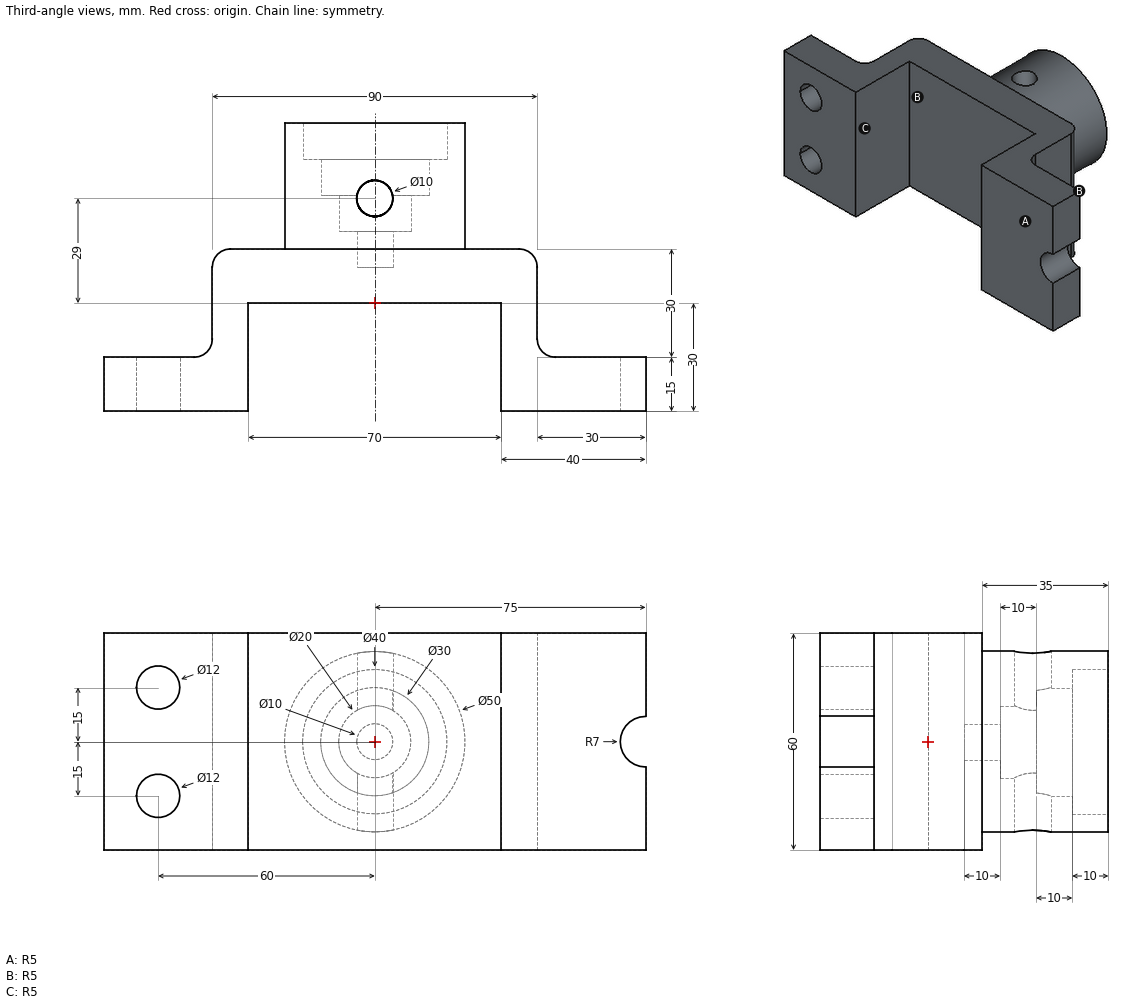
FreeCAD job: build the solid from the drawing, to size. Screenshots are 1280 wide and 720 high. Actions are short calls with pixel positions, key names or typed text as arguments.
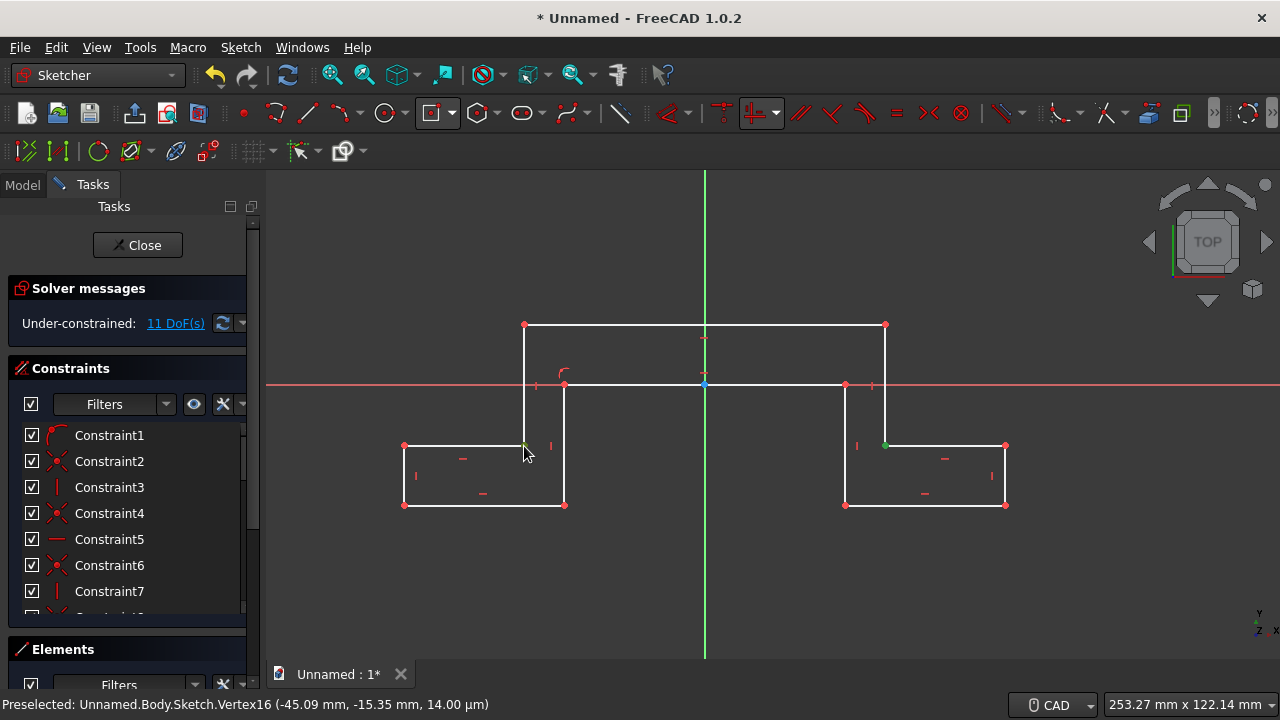
click(705, 600)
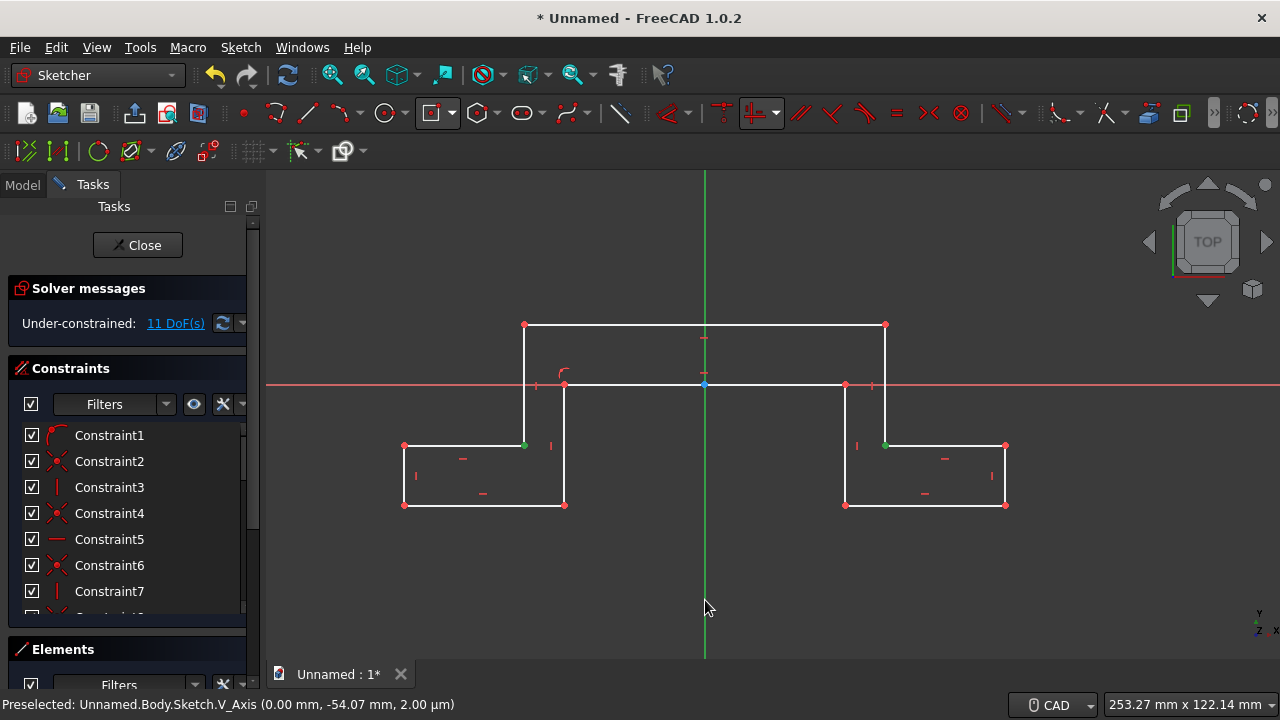
click(930, 114)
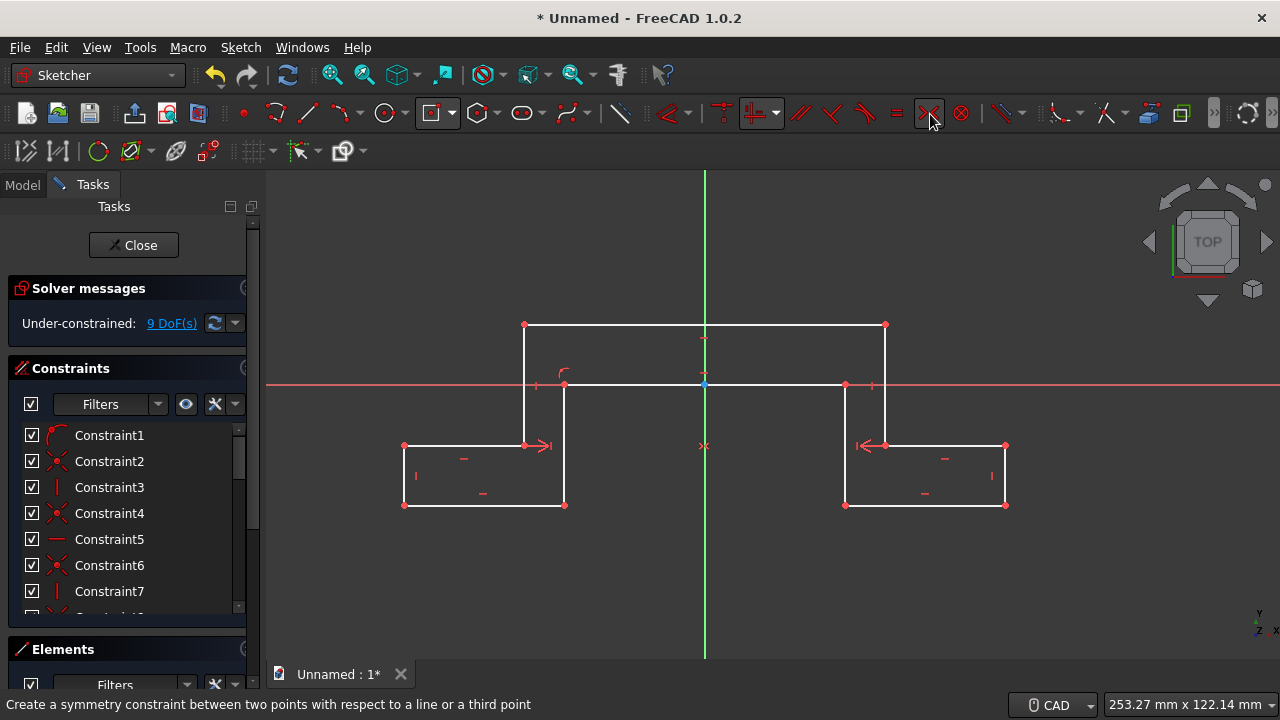
click(1005, 506)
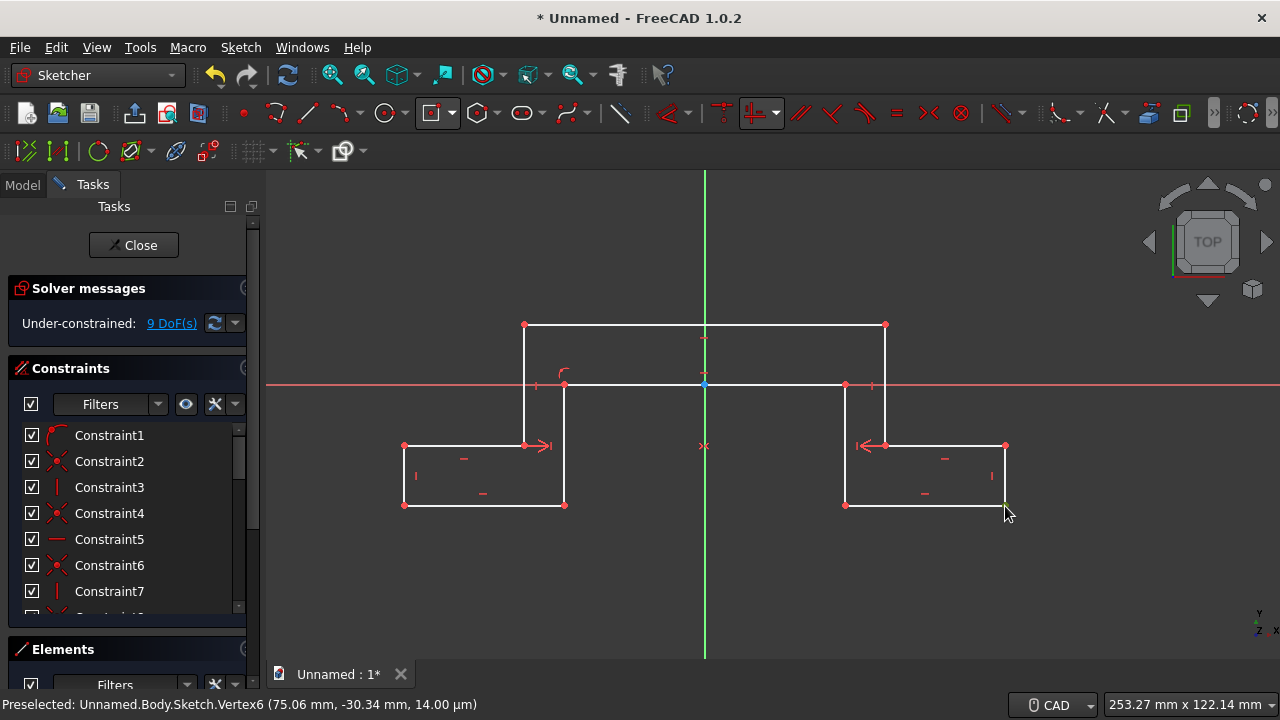
click(404, 506)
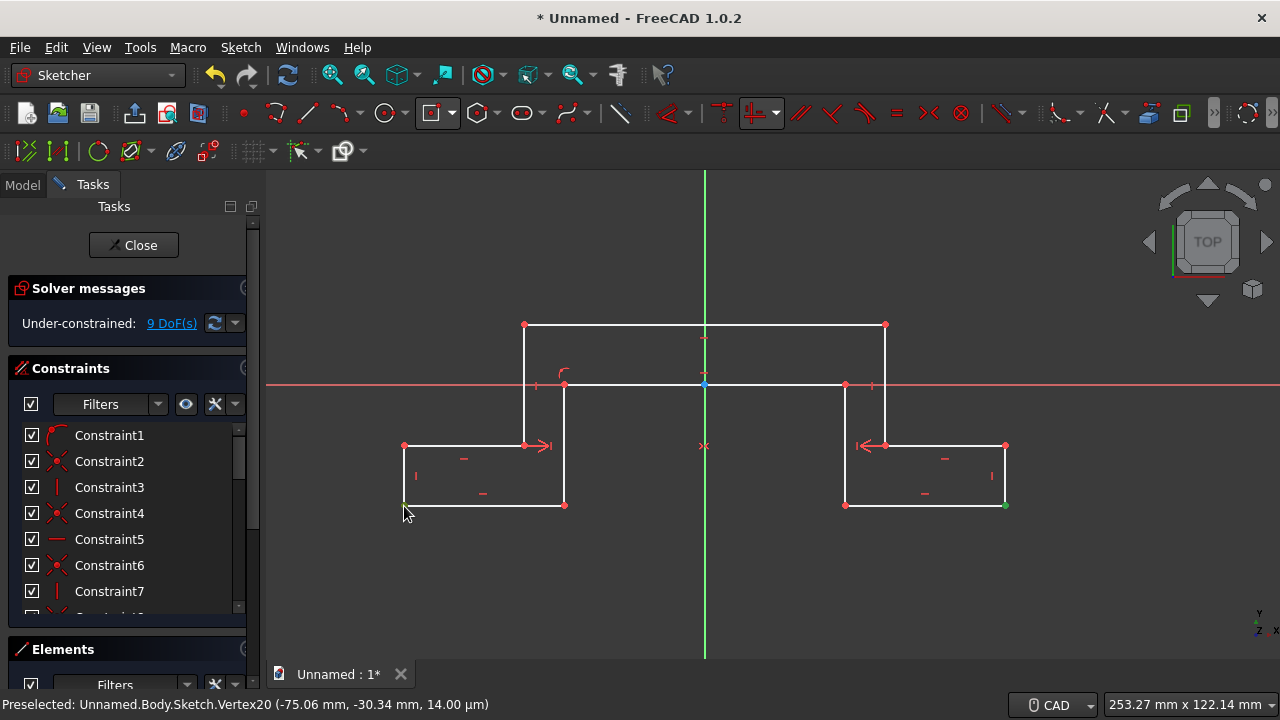
click(705, 600)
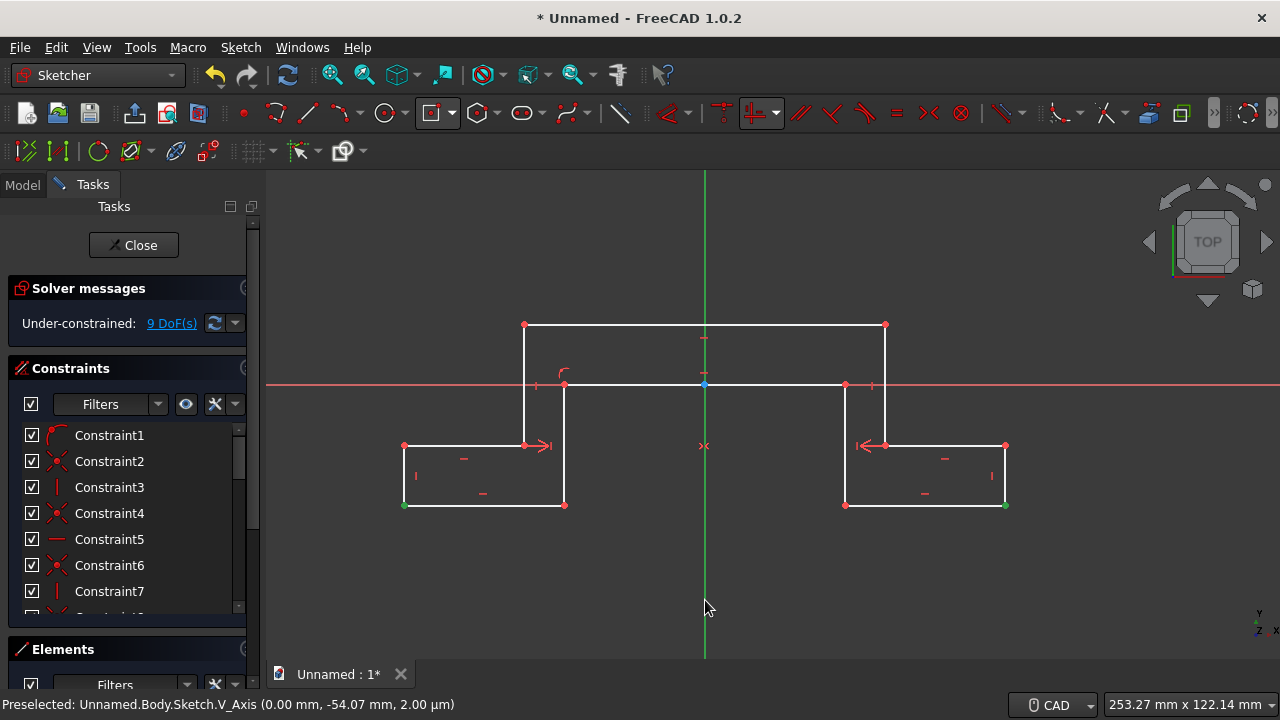
click(930, 114)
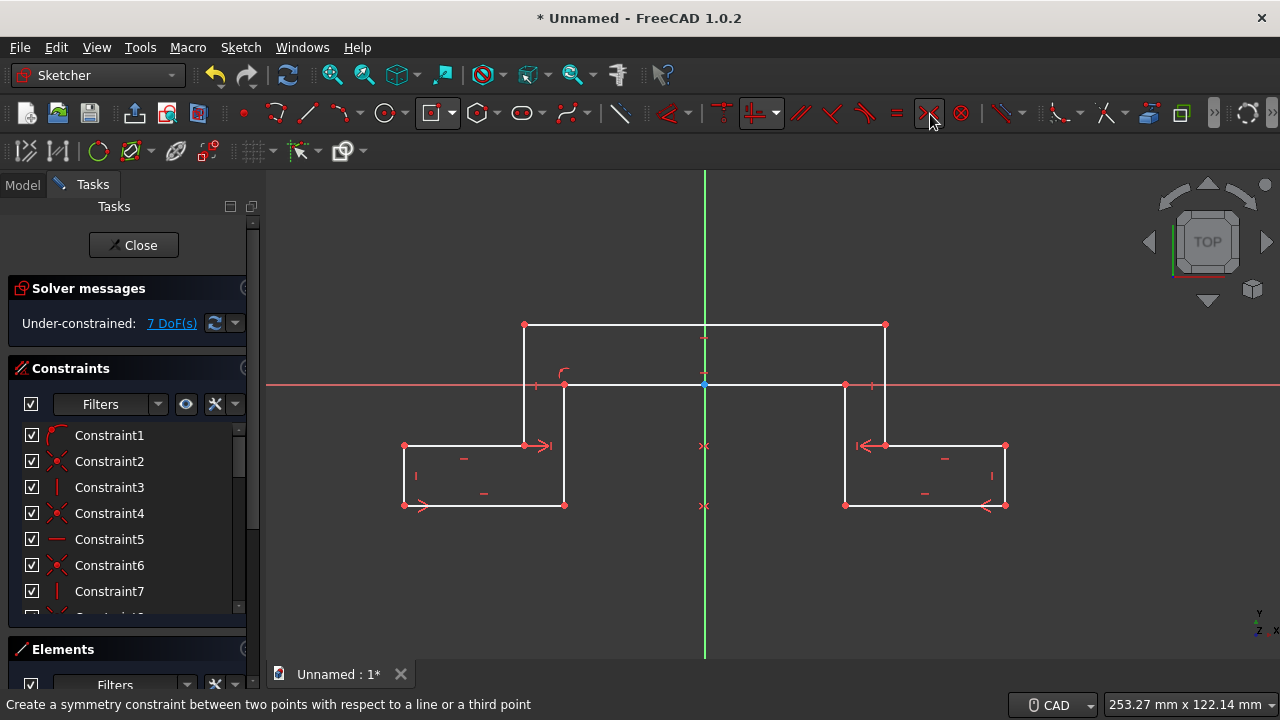
click(668, 114)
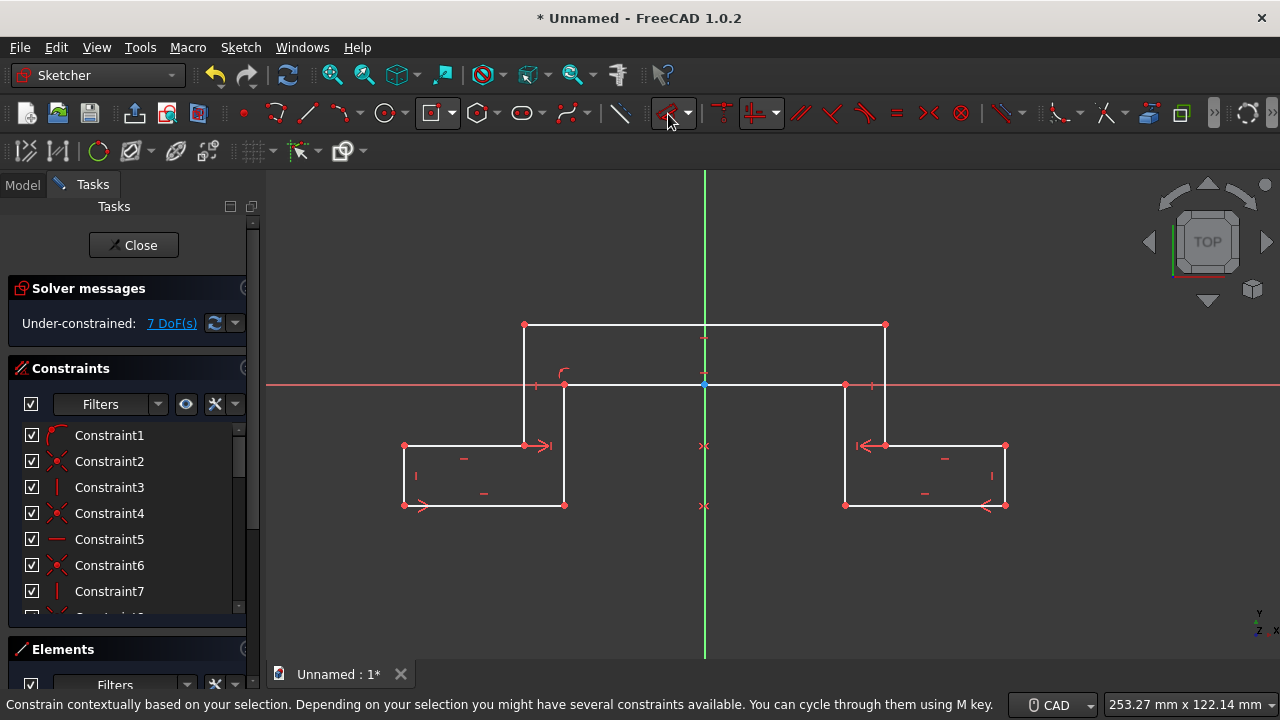
click(648, 385)
click(640, 351)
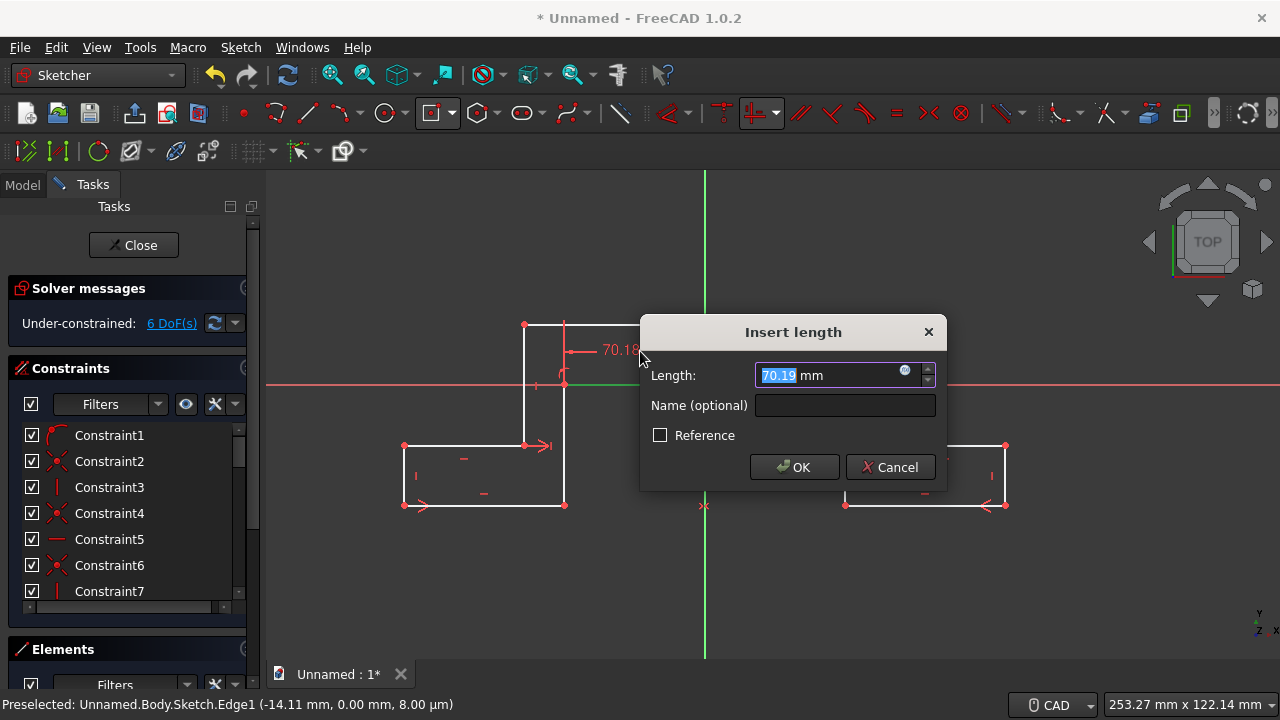
text(70)
key(Return)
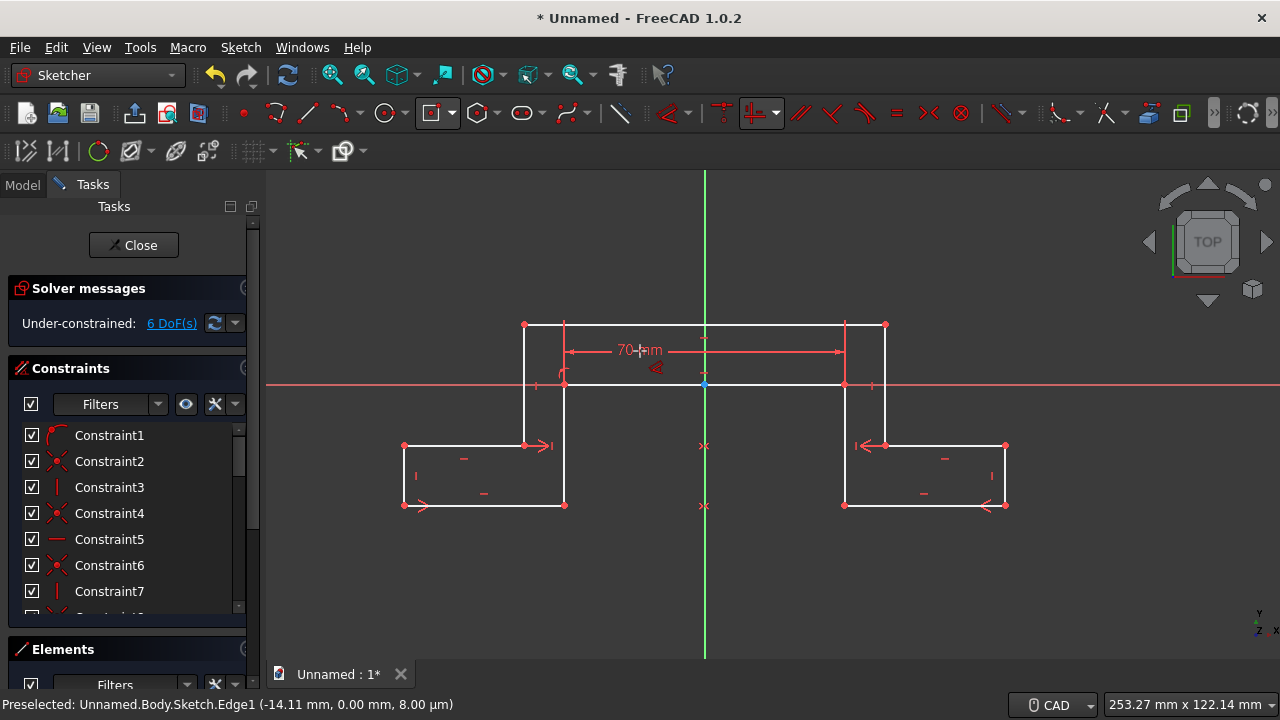
click(845, 421)
click(879, 473)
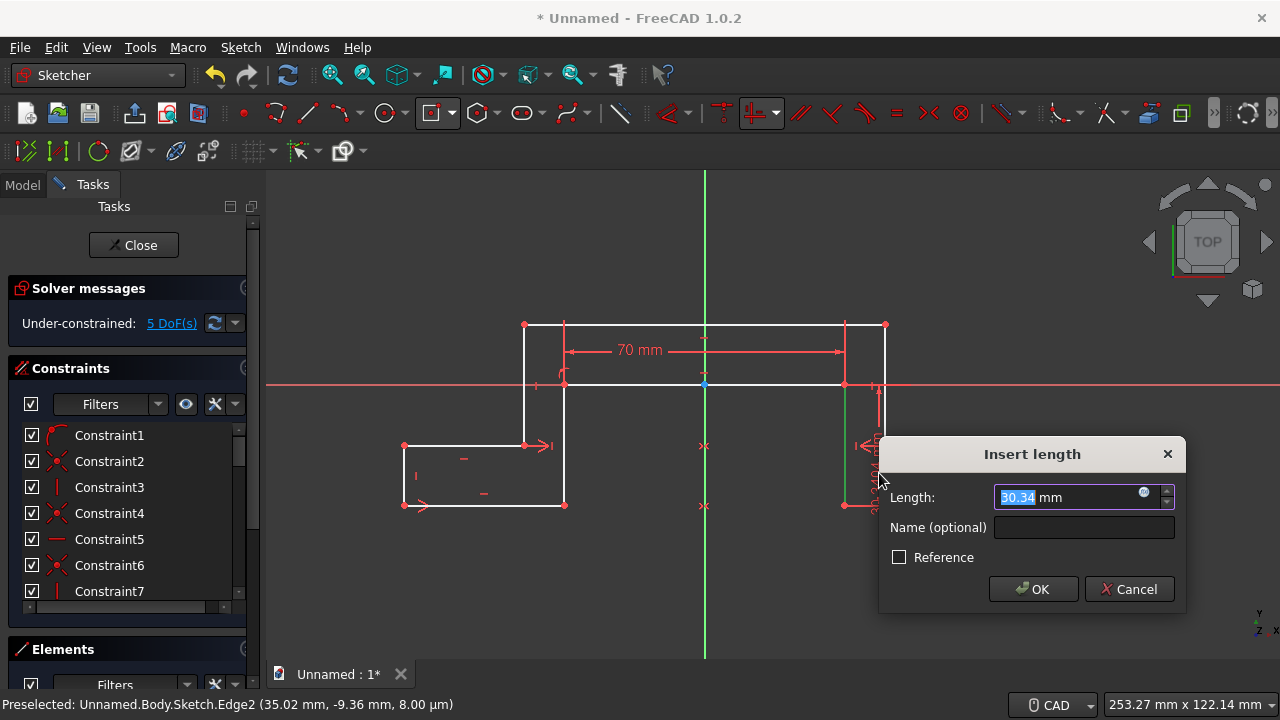
text(30)
key(Return)